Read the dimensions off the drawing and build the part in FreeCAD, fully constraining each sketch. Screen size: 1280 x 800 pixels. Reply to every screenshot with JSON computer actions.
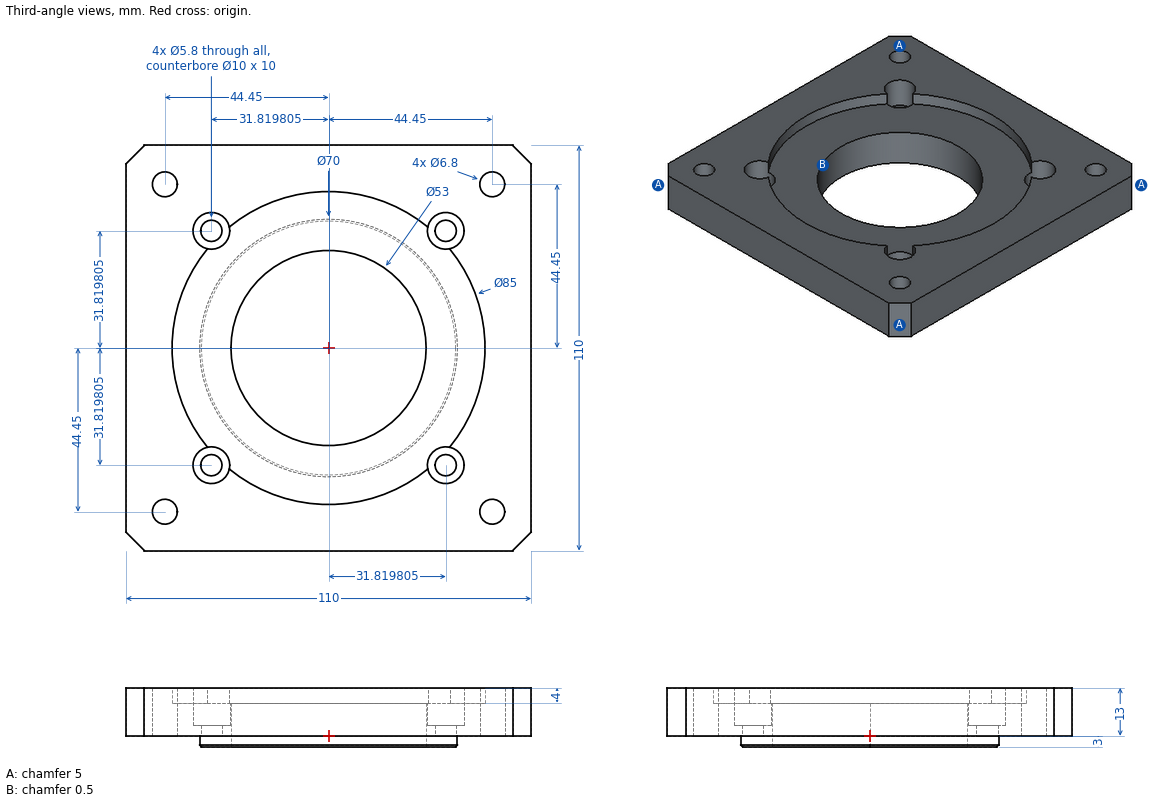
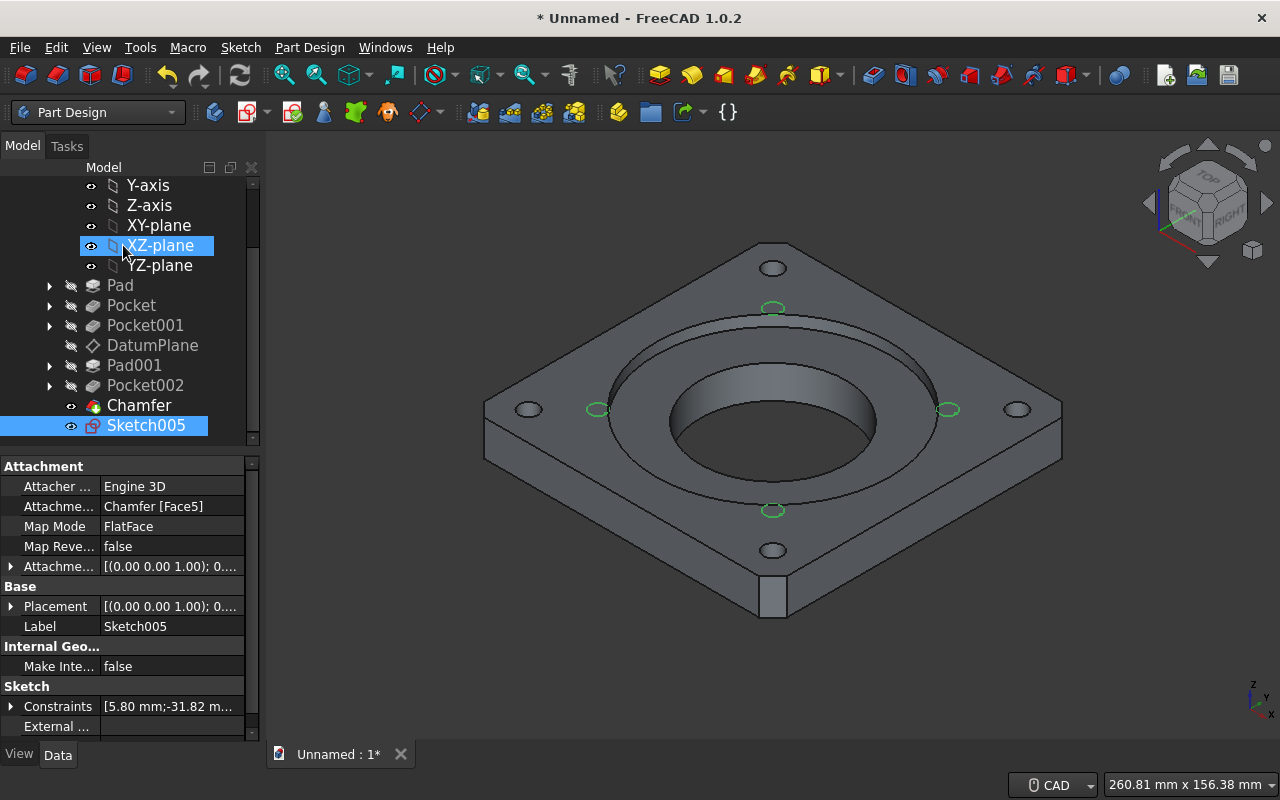
{"action": "left_click", "coordinate": [906, 76]}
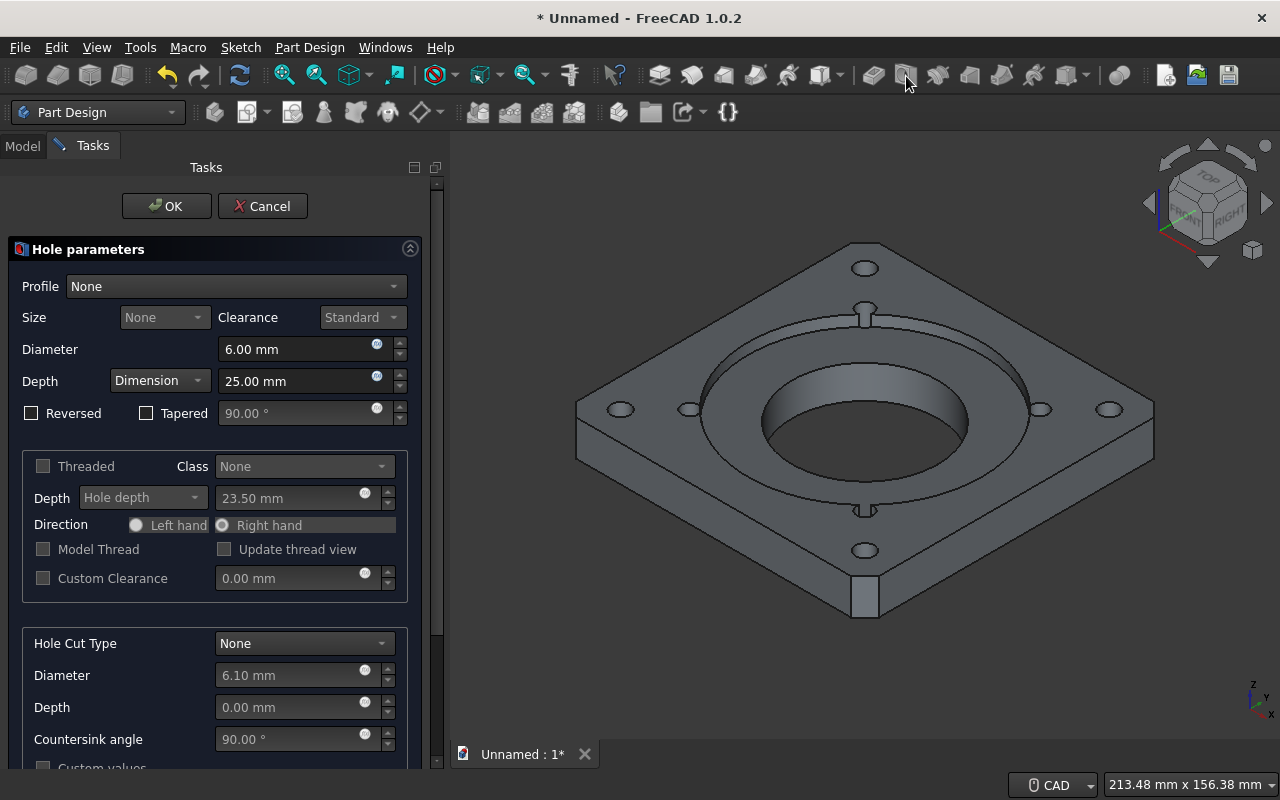
{"action": "triple_click", "coordinate": [305, 349]}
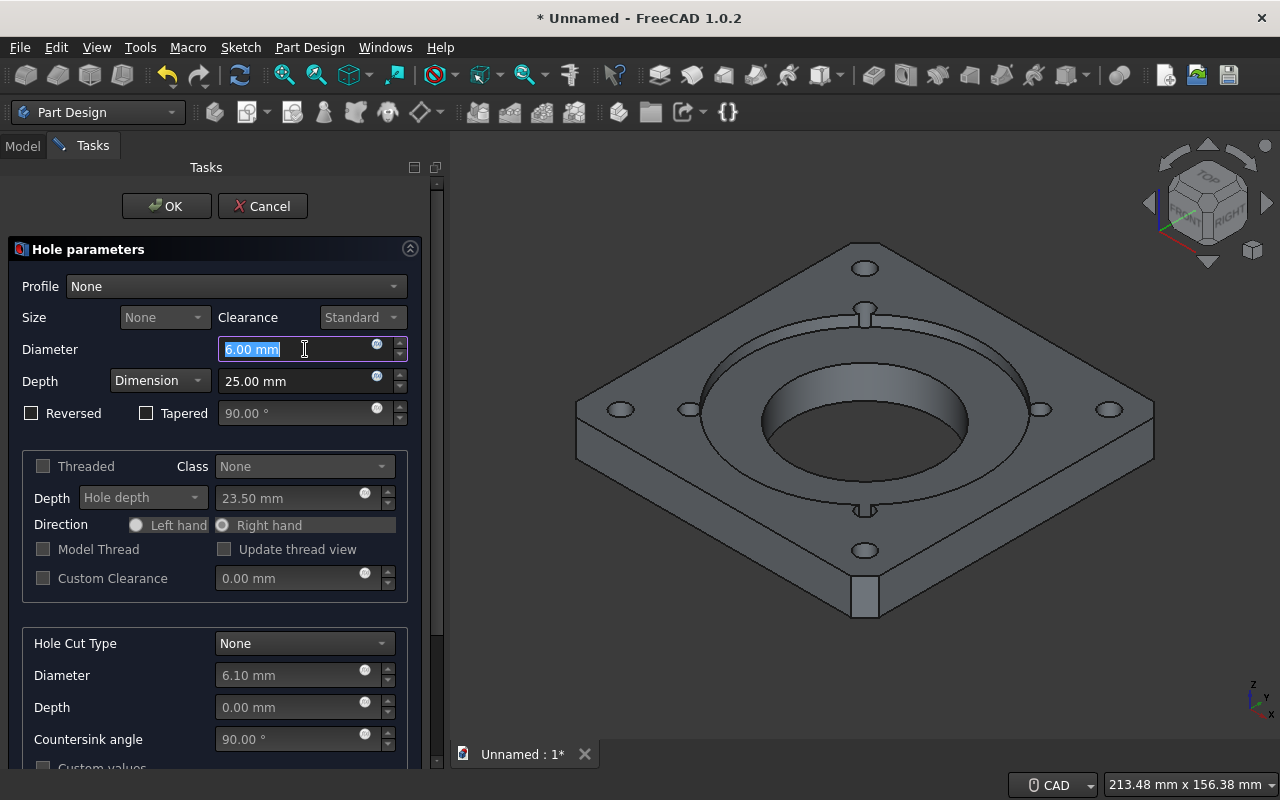
{"action": "type", "text": "5.8"}
{"action": "key", "text": "Tab"}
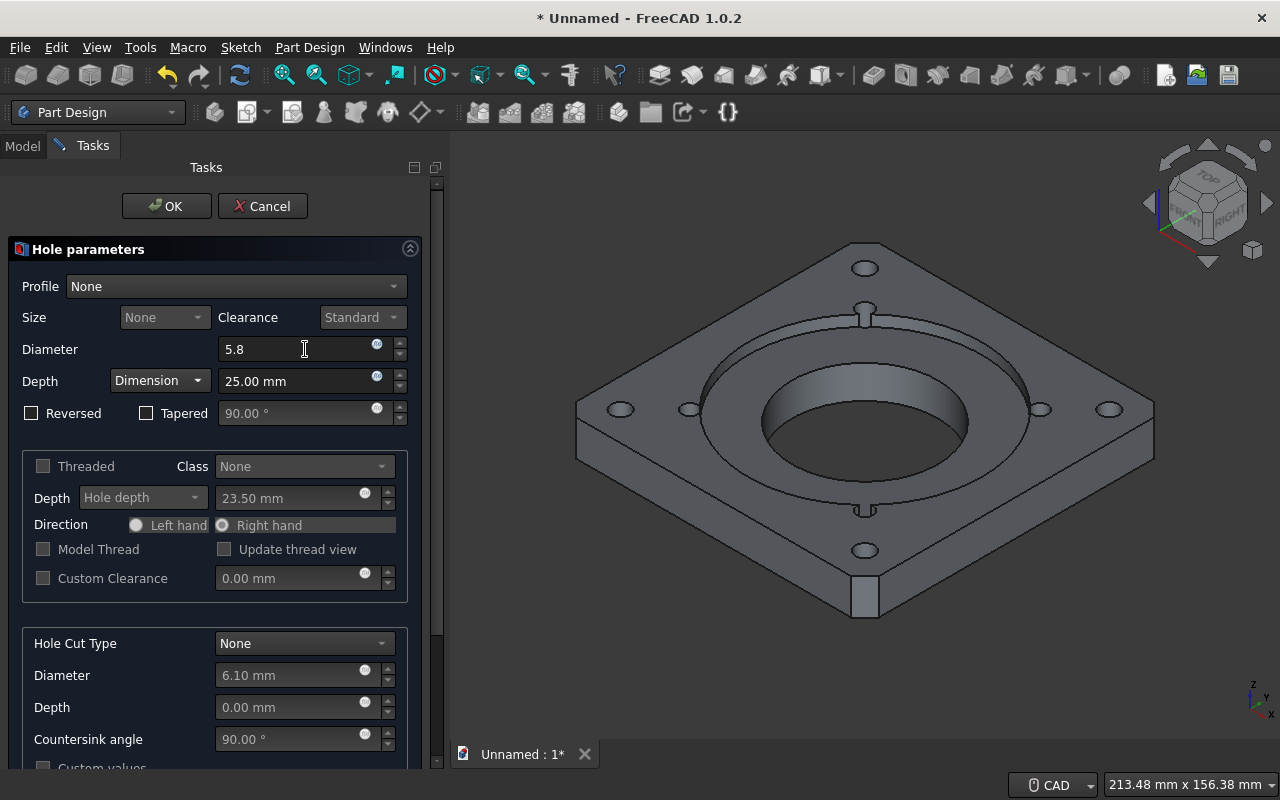
{"action": "left_click", "coordinate": [161, 380]}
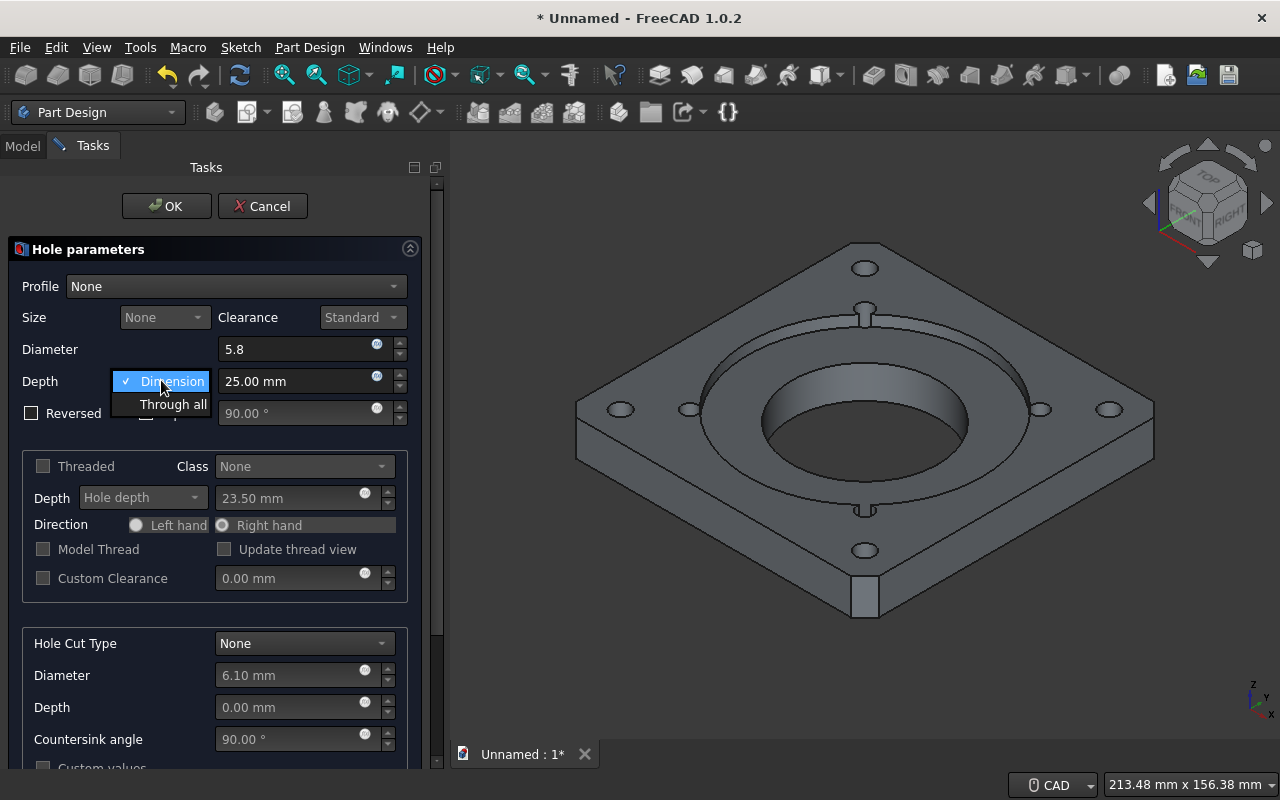
{"action": "left_click", "coordinate": [160, 404]}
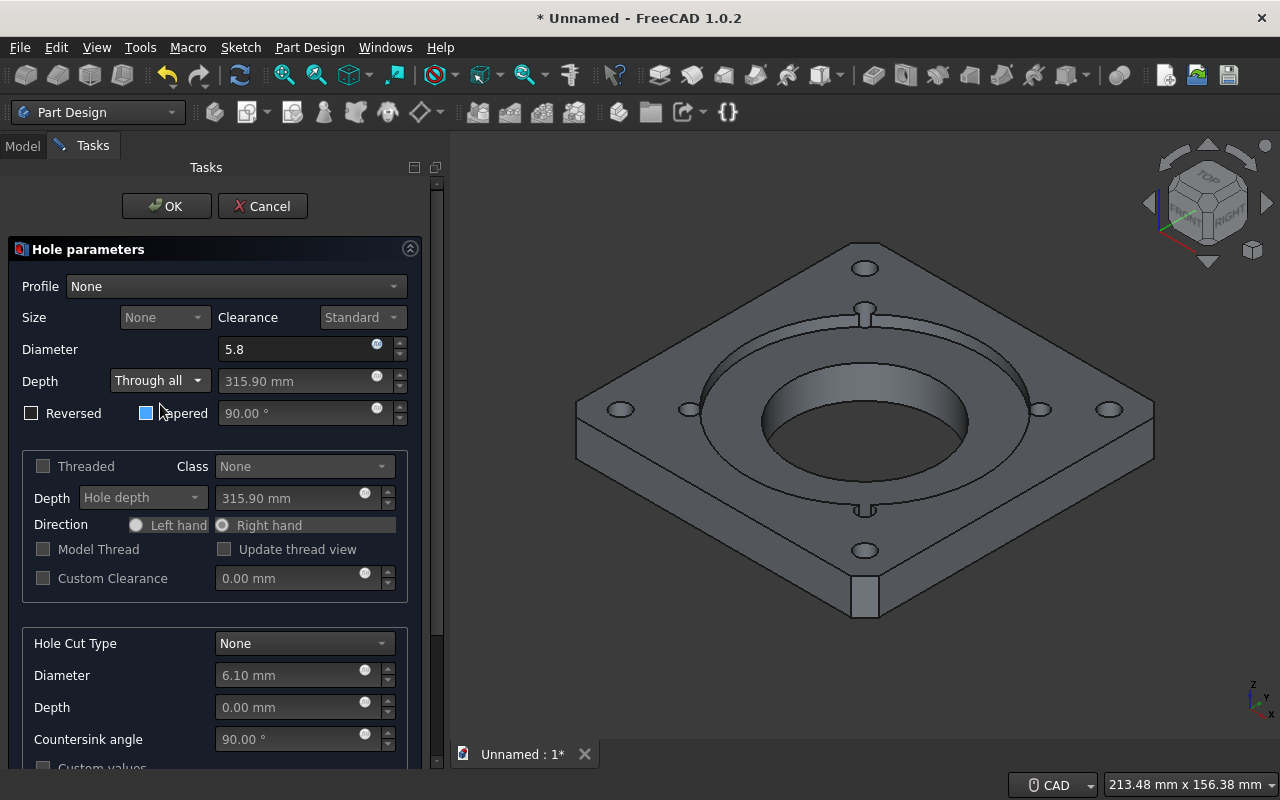
{"action": "left_click", "coordinate": [306, 644]}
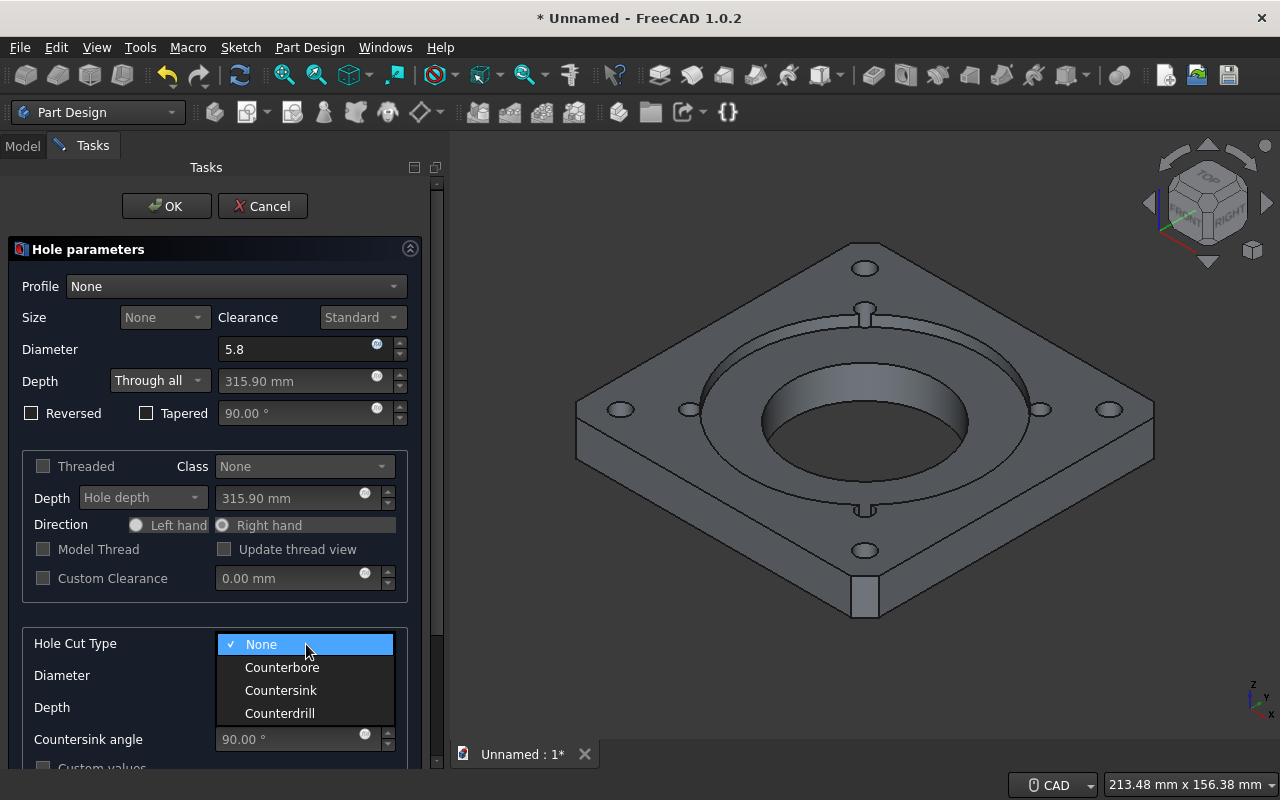
{"action": "left_click", "coordinate": [304, 668]}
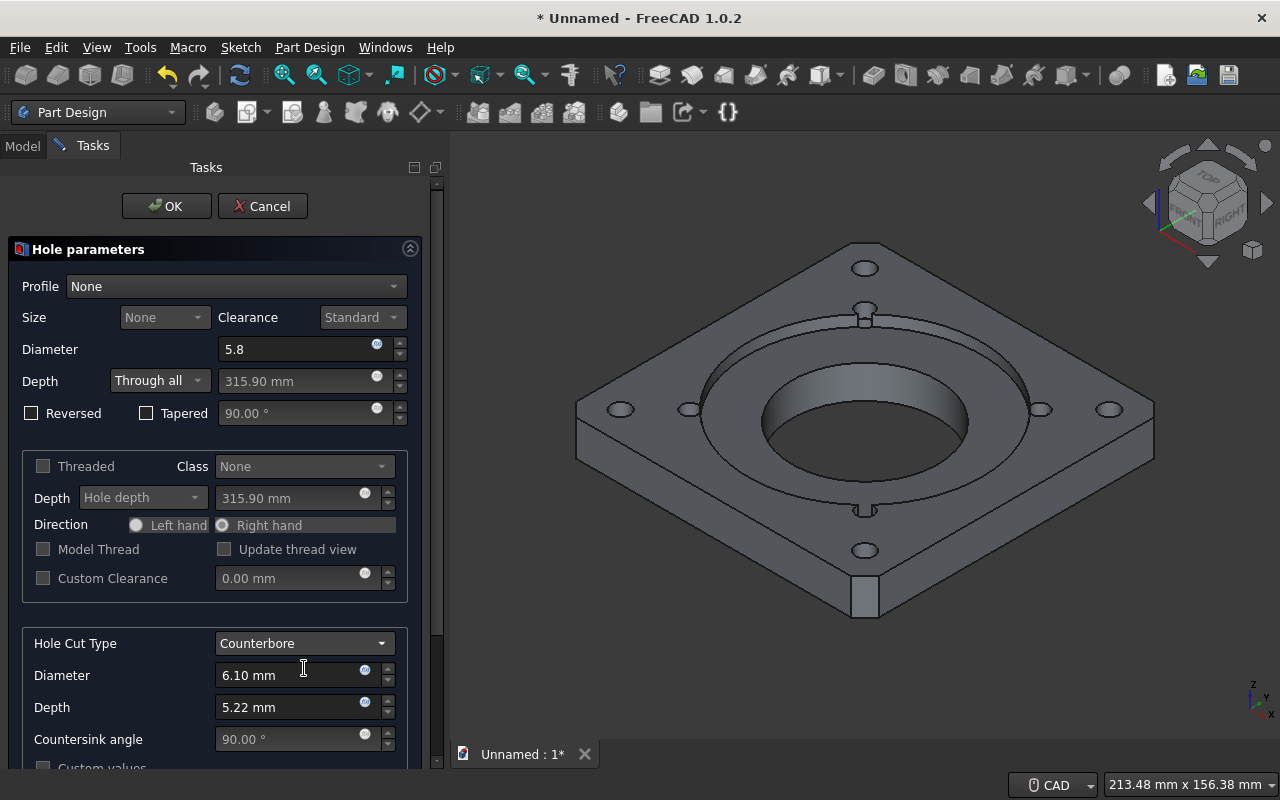
{"action": "triple_click", "coordinate": [298, 675]}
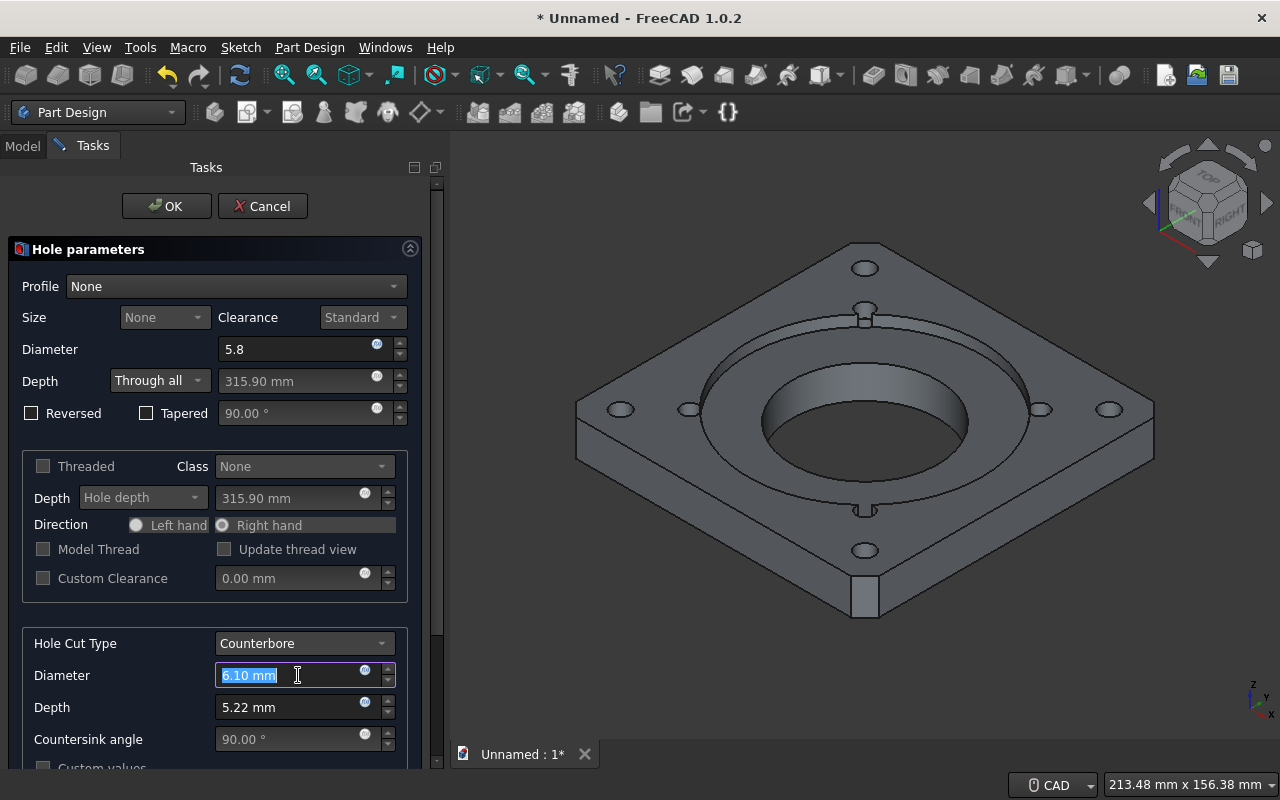
{"action": "type", "text": "10"}
{"action": "key", "text": "Tab"}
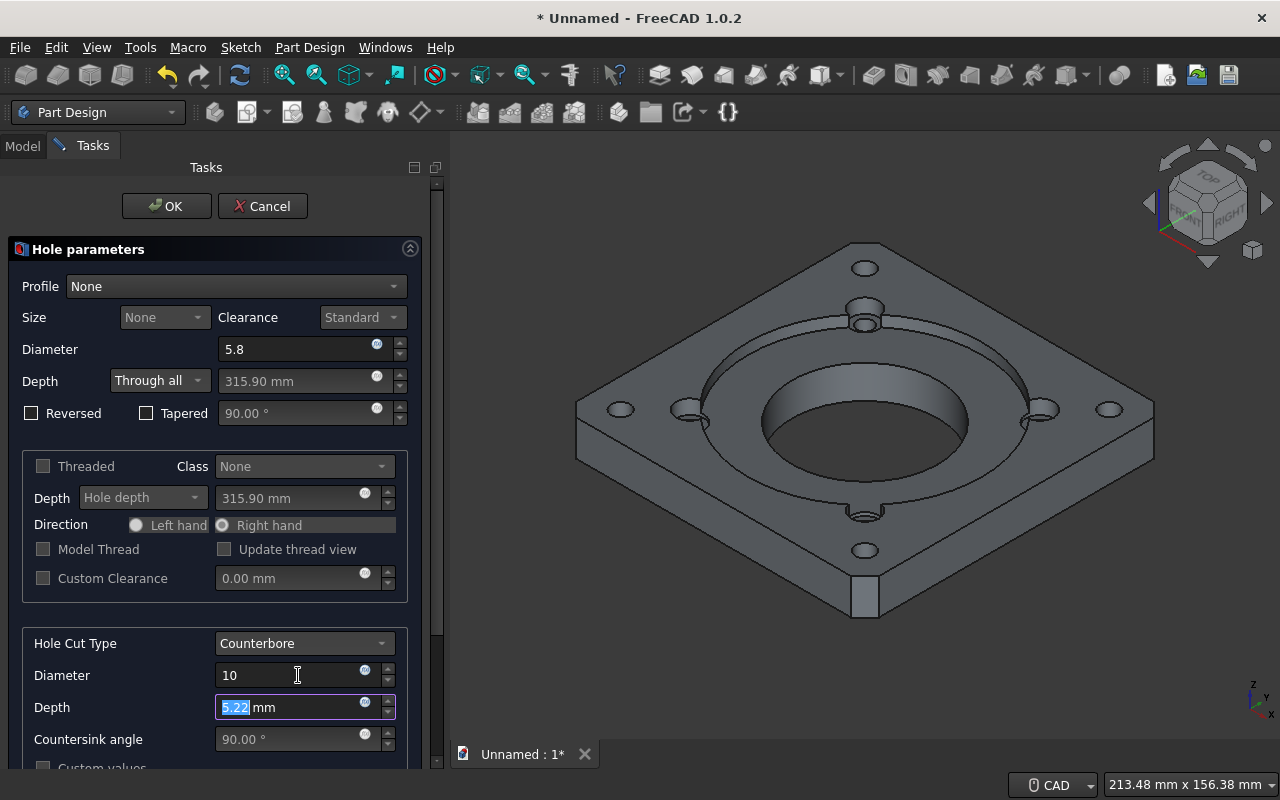
{"action": "type", "text": "10"}
{"action": "key", "text": "Tab"}